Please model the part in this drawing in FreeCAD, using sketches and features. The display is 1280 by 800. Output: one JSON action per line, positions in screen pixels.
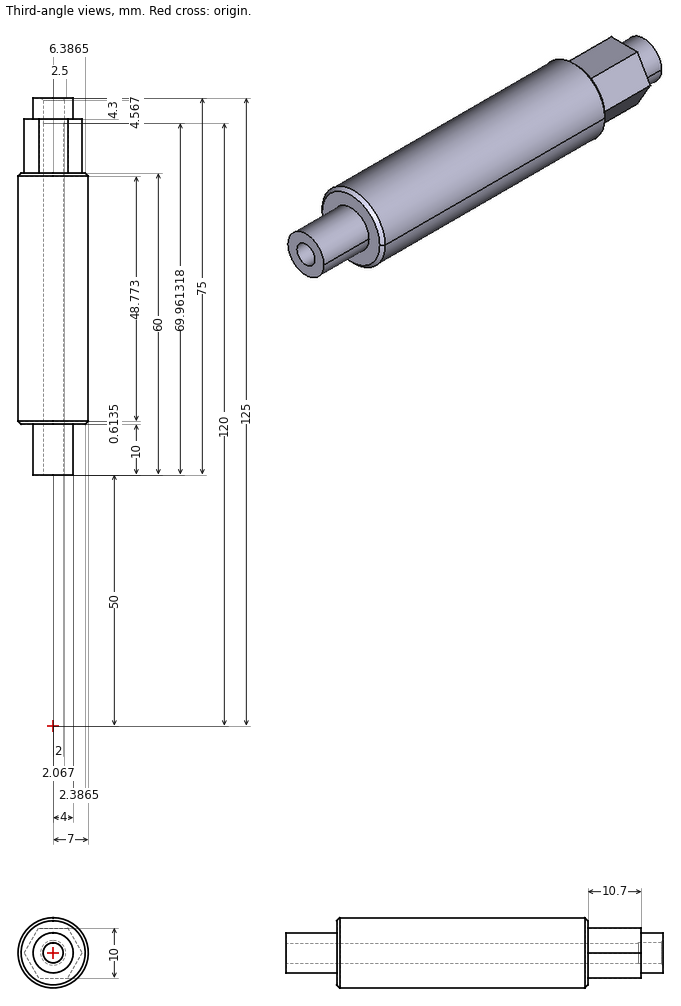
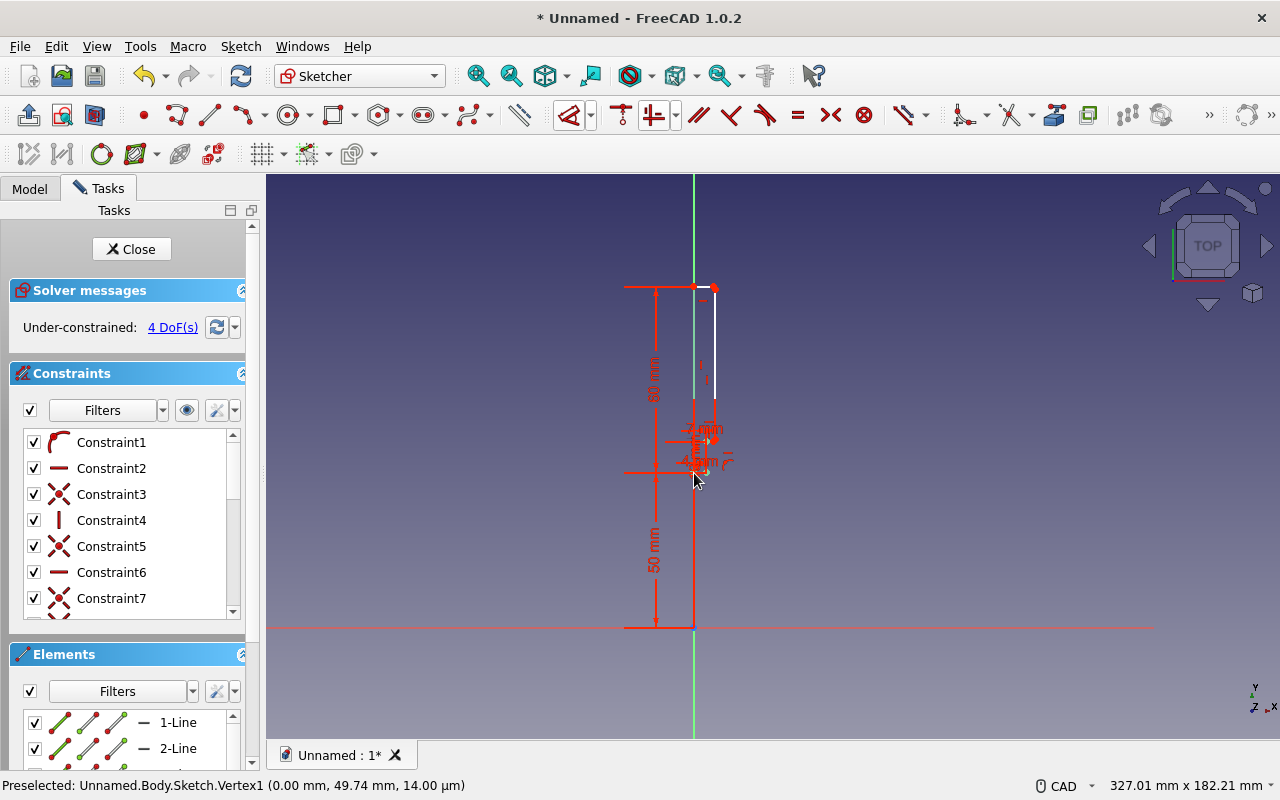
{"action": "scroll", "coordinate": [710, 442], "scroll_direction": "up", "scroll_amount": 9}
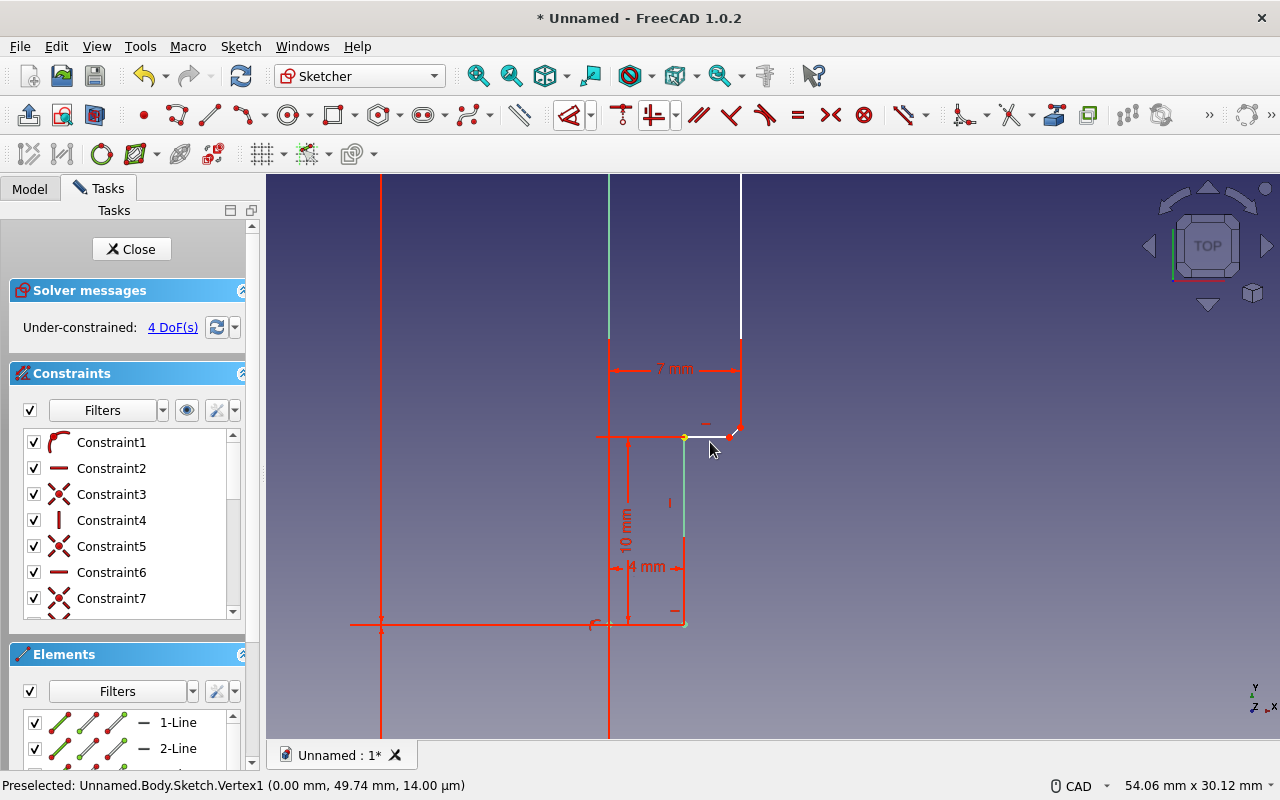
{"action": "left_click", "coordinate": [707, 437]}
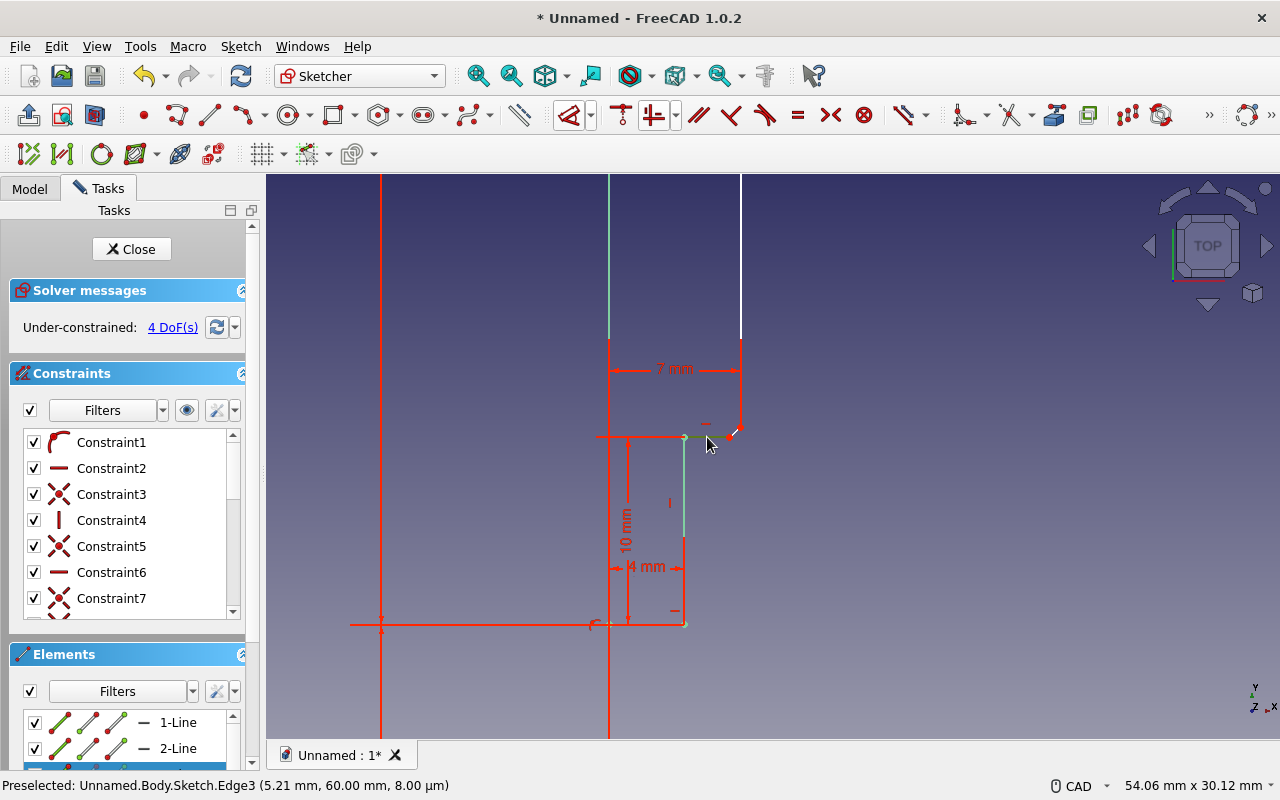
{"action": "key", "text": "l"}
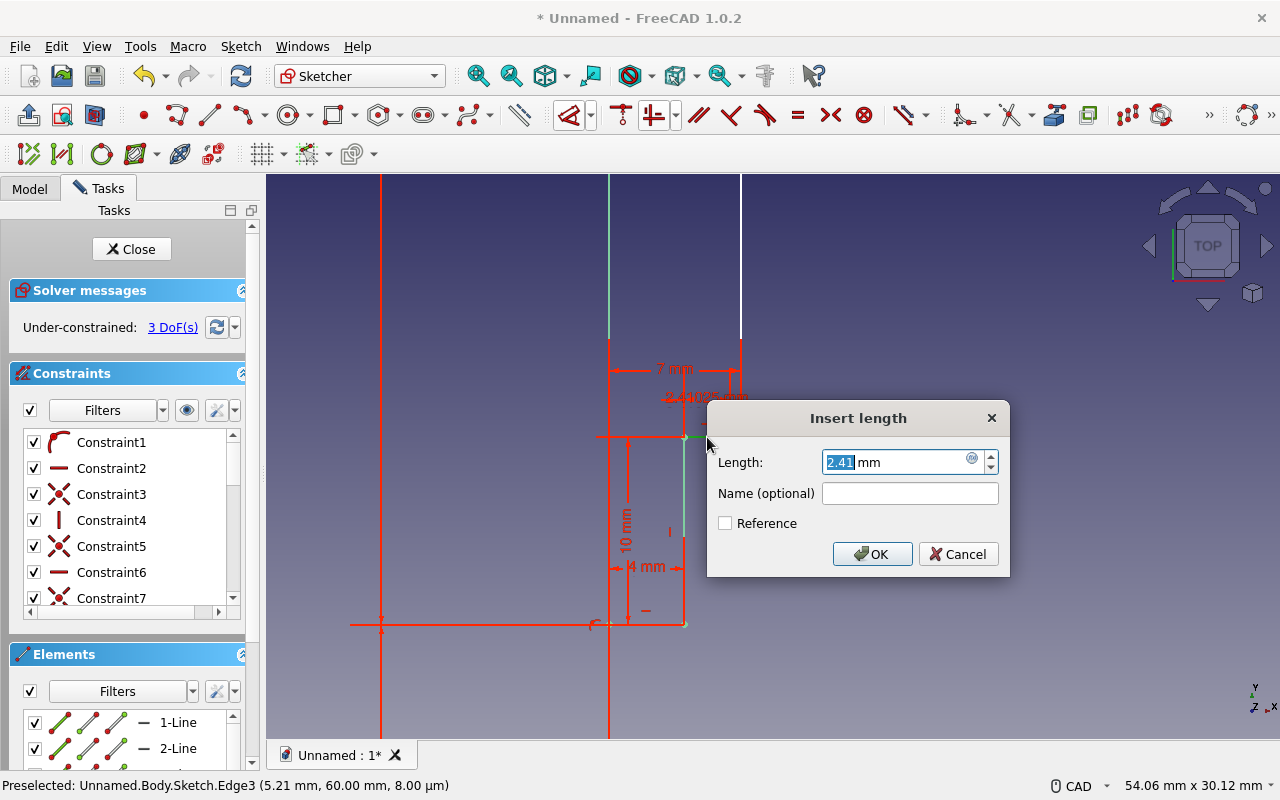
{"action": "type", "text": "2.3865"}
{"action": "key", "text": "Return"}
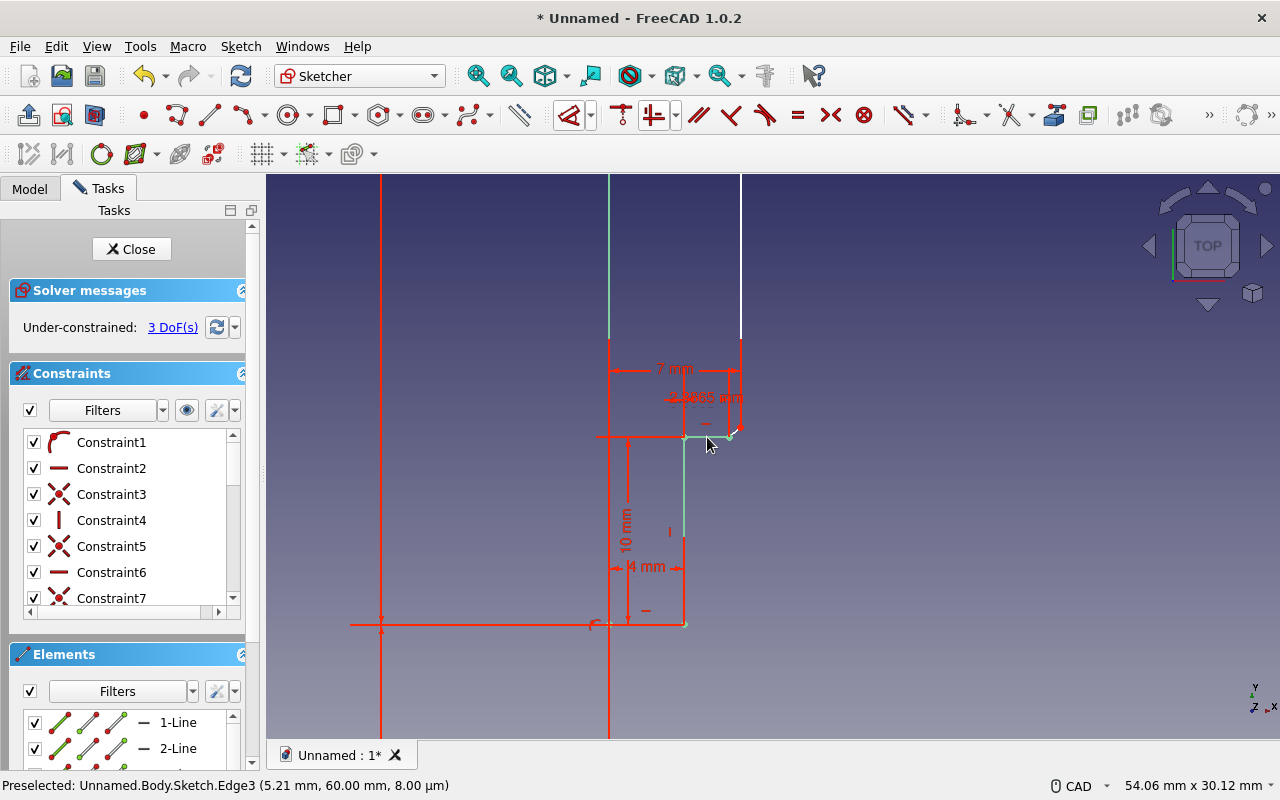
{"action": "scroll", "coordinate": [710, 442], "scroll_direction": "down", "scroll_amount": 9}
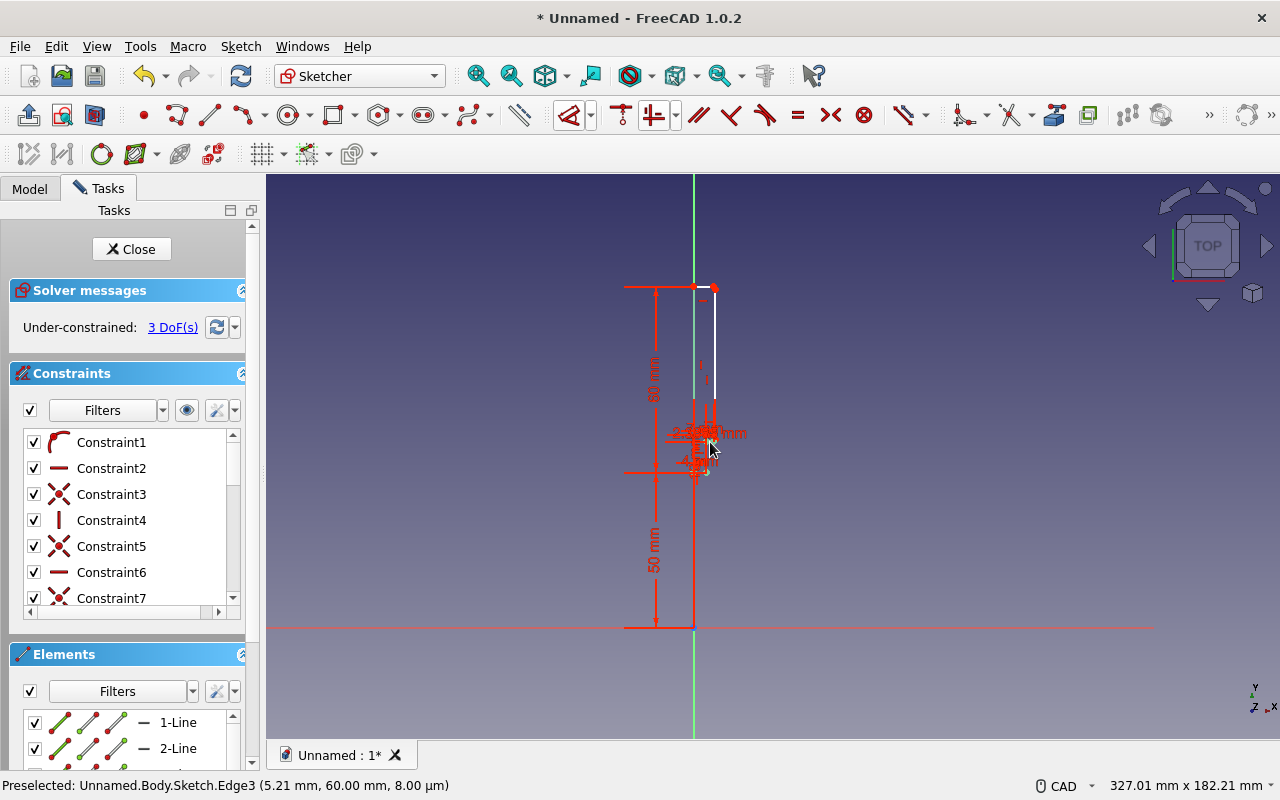
{"action": "left_click", "coordinate": [715, 410]}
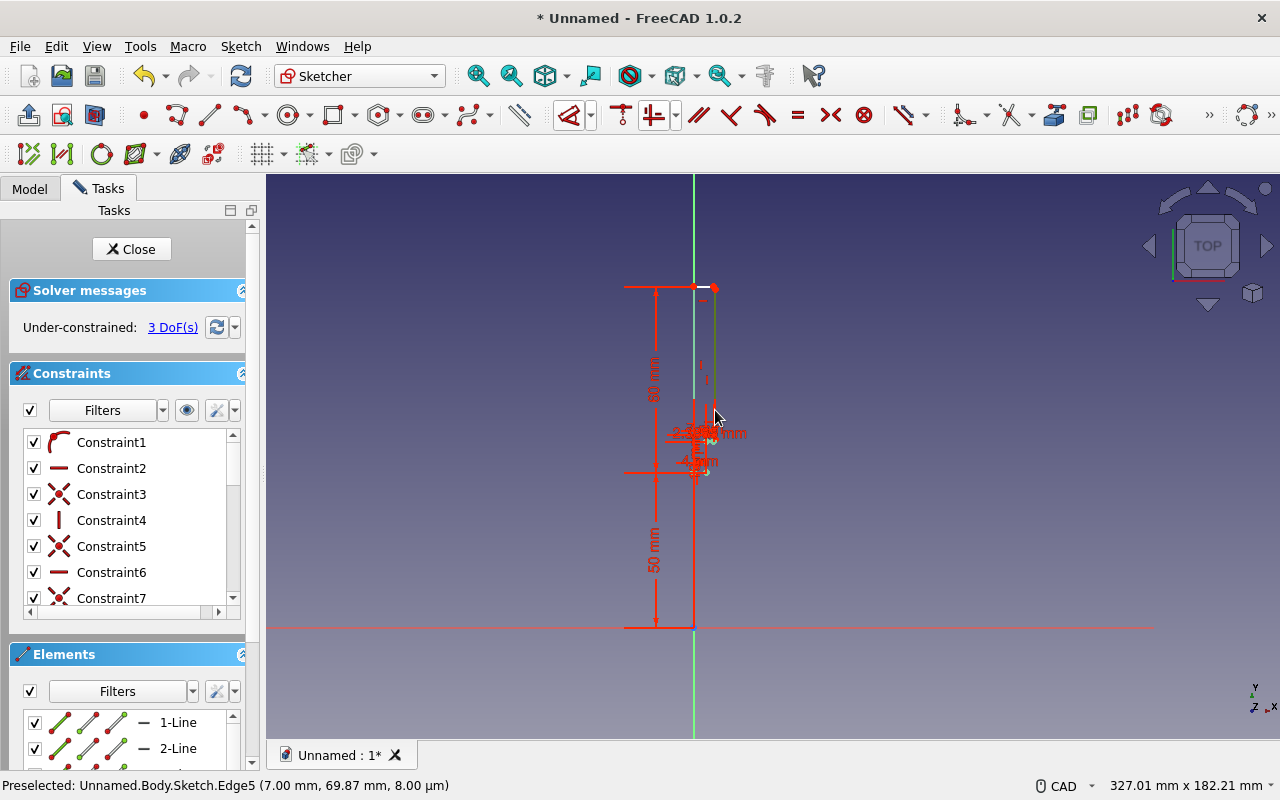
{"action": "key", "text": "i"}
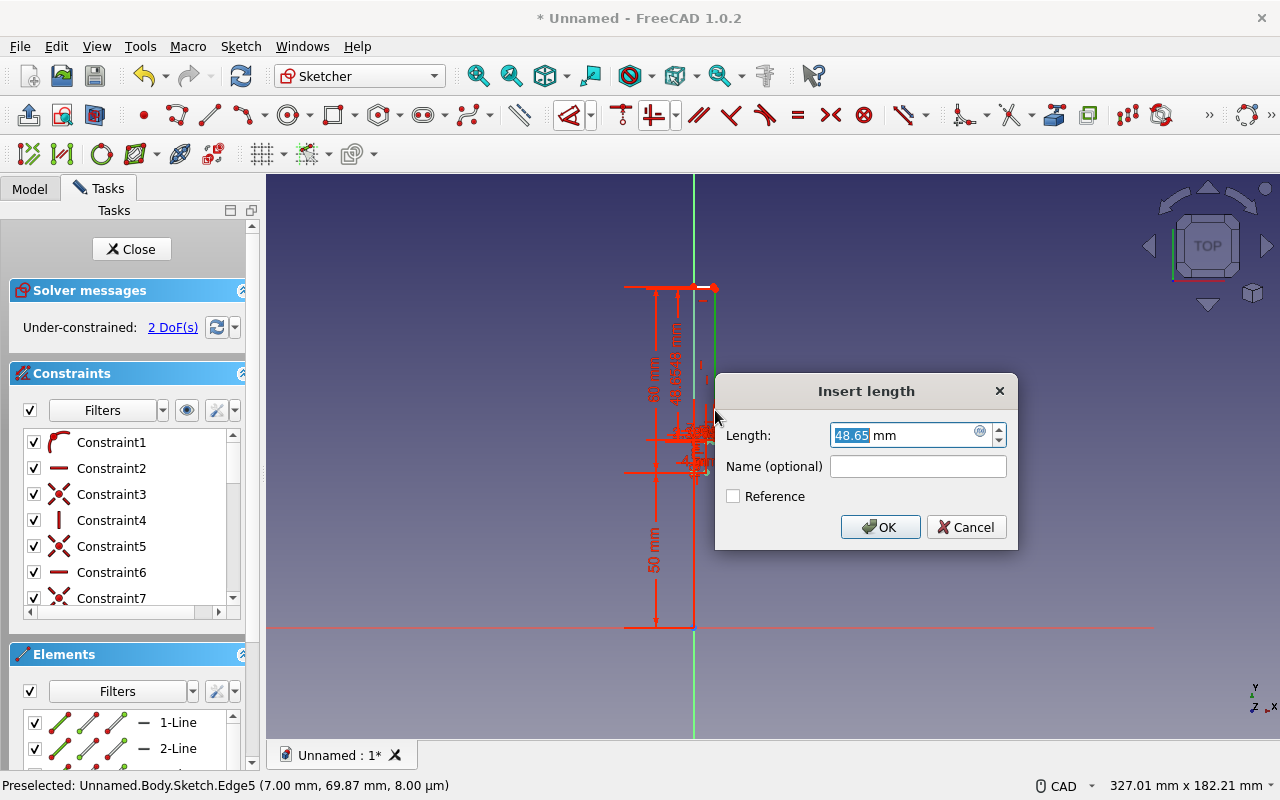
{"action": "type", "text": "48.773"}
{"action": "key", "text": "Return"}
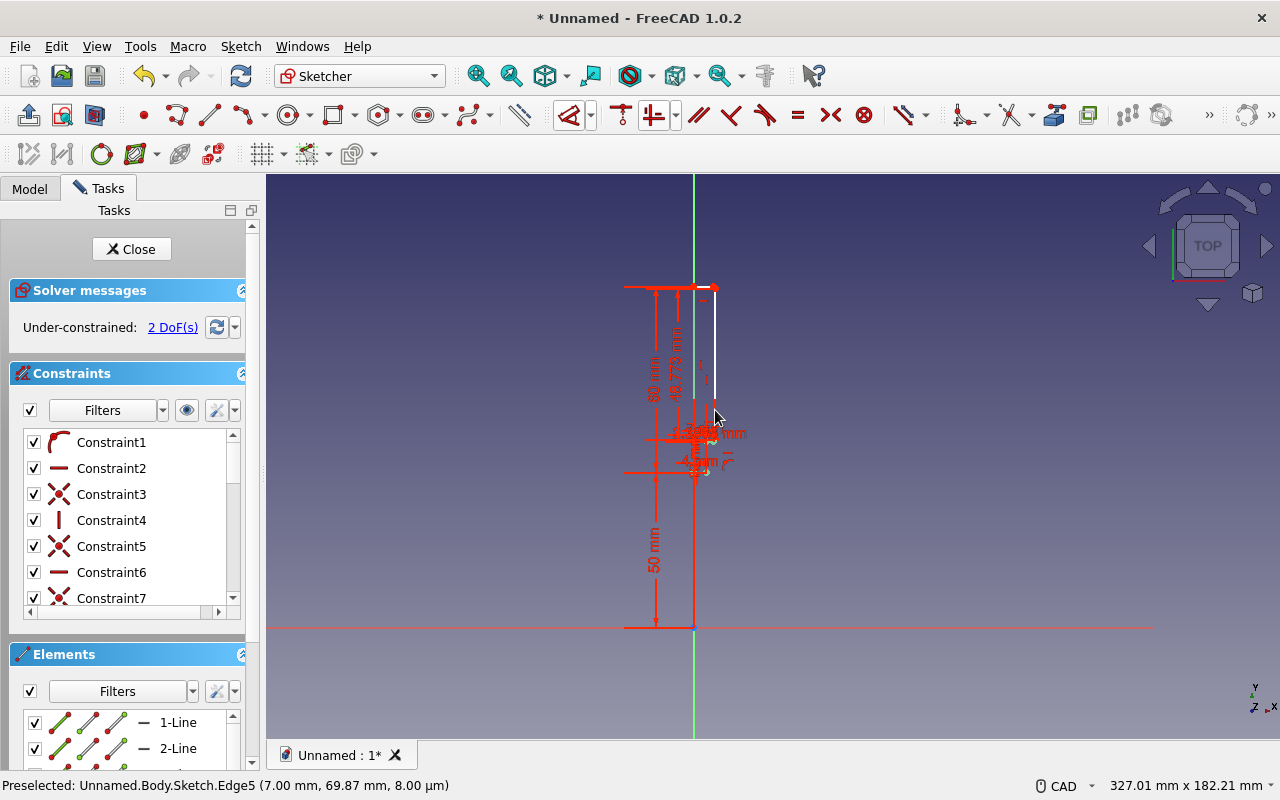
{"action": "scroll", "coordinate": [704, 287], "scroll_direction": "up", "scroll_amount": 4}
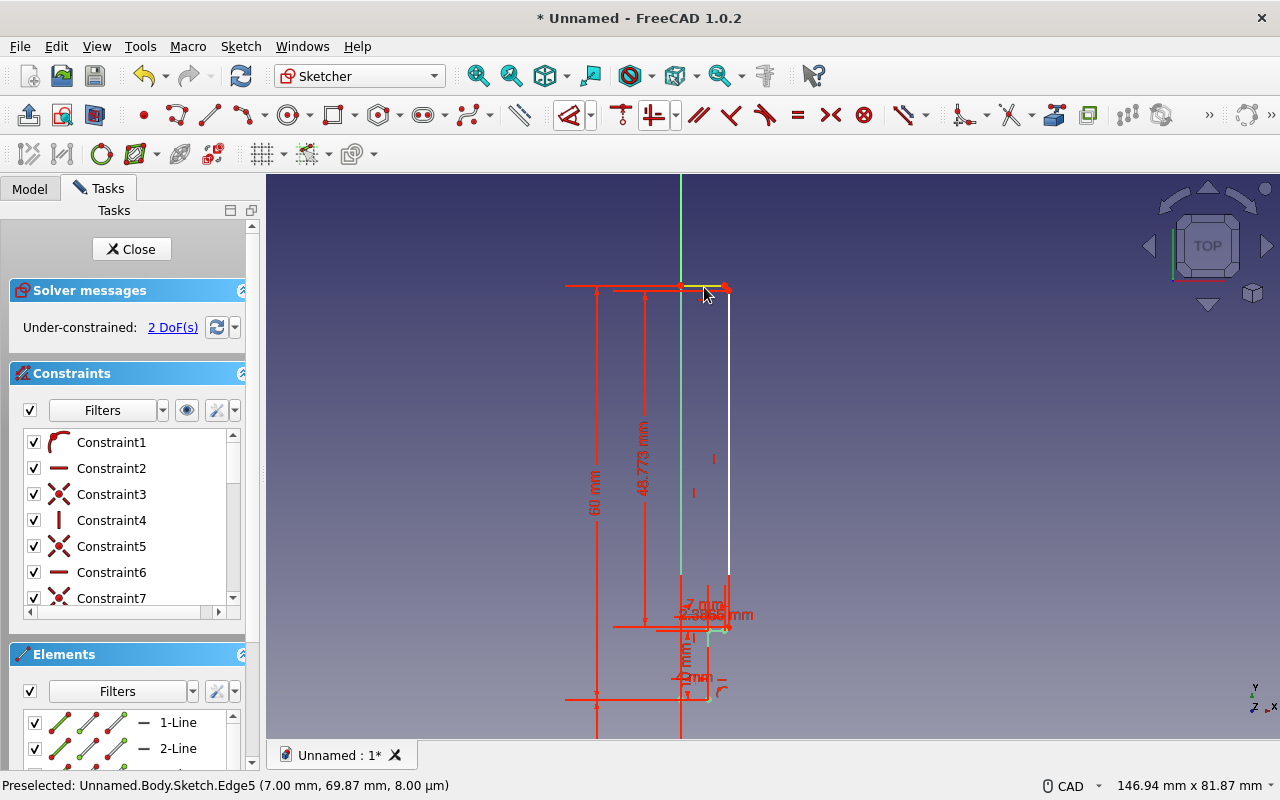
{"action": "left_click", "coordinate": [703, 286]}